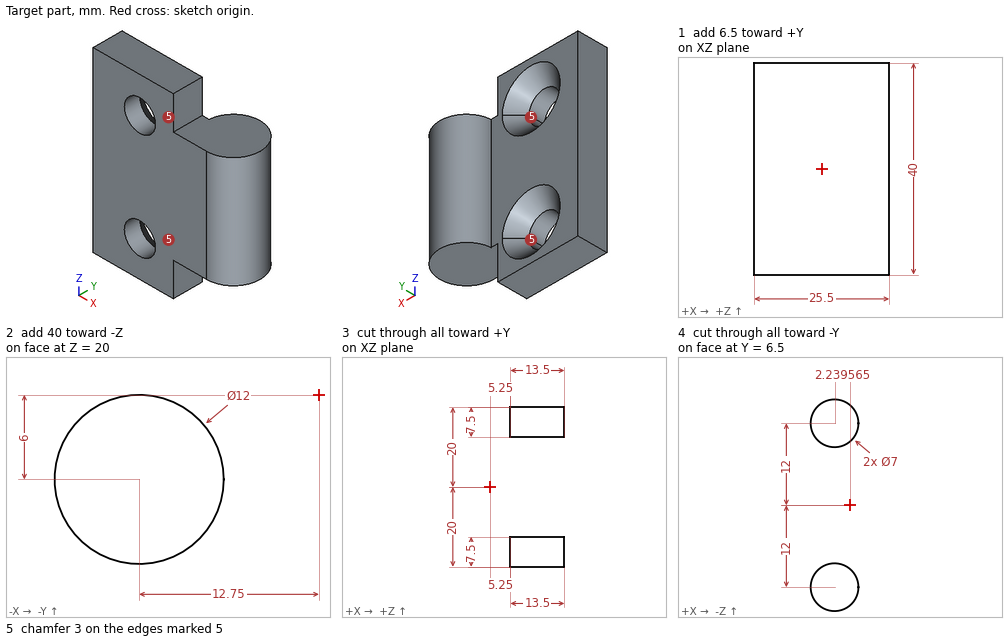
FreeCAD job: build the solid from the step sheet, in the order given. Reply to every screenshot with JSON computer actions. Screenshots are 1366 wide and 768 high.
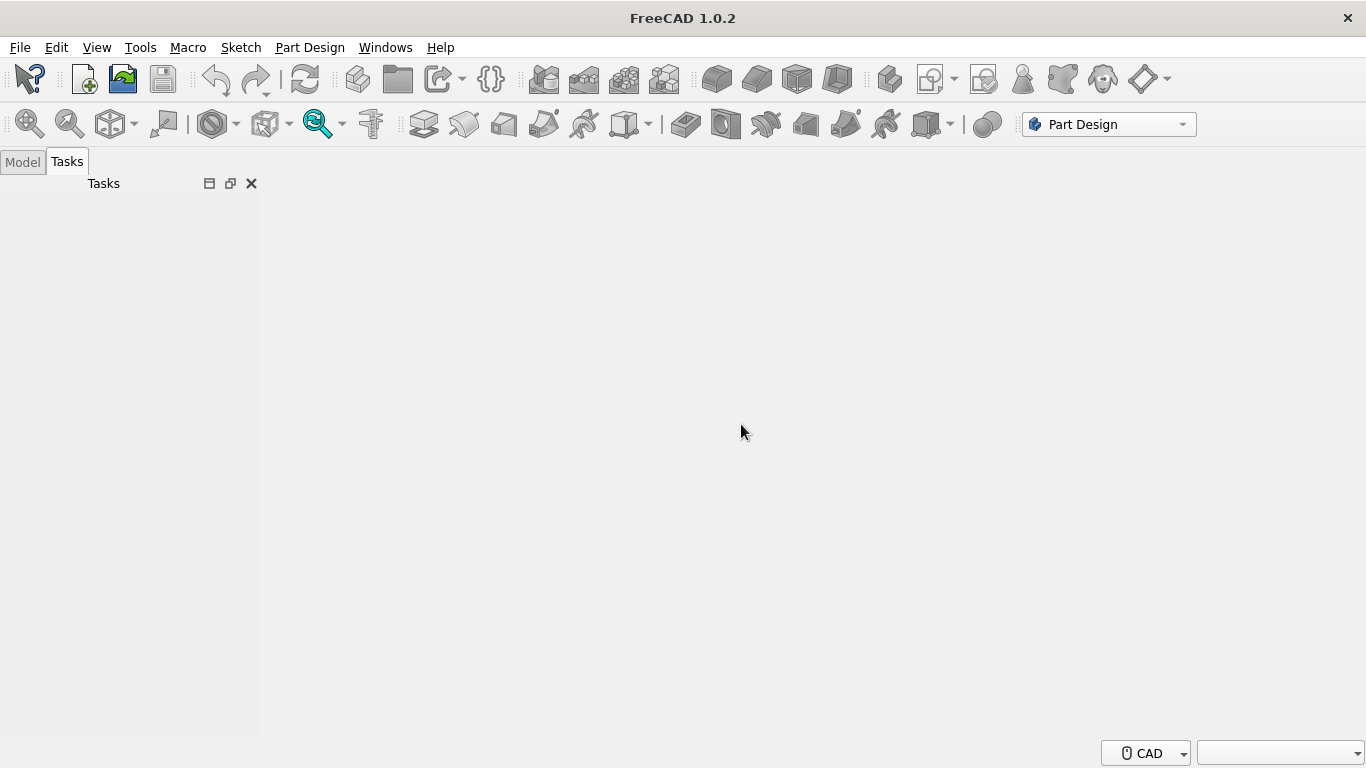
{"action": "key", "text": "ctrl+n"}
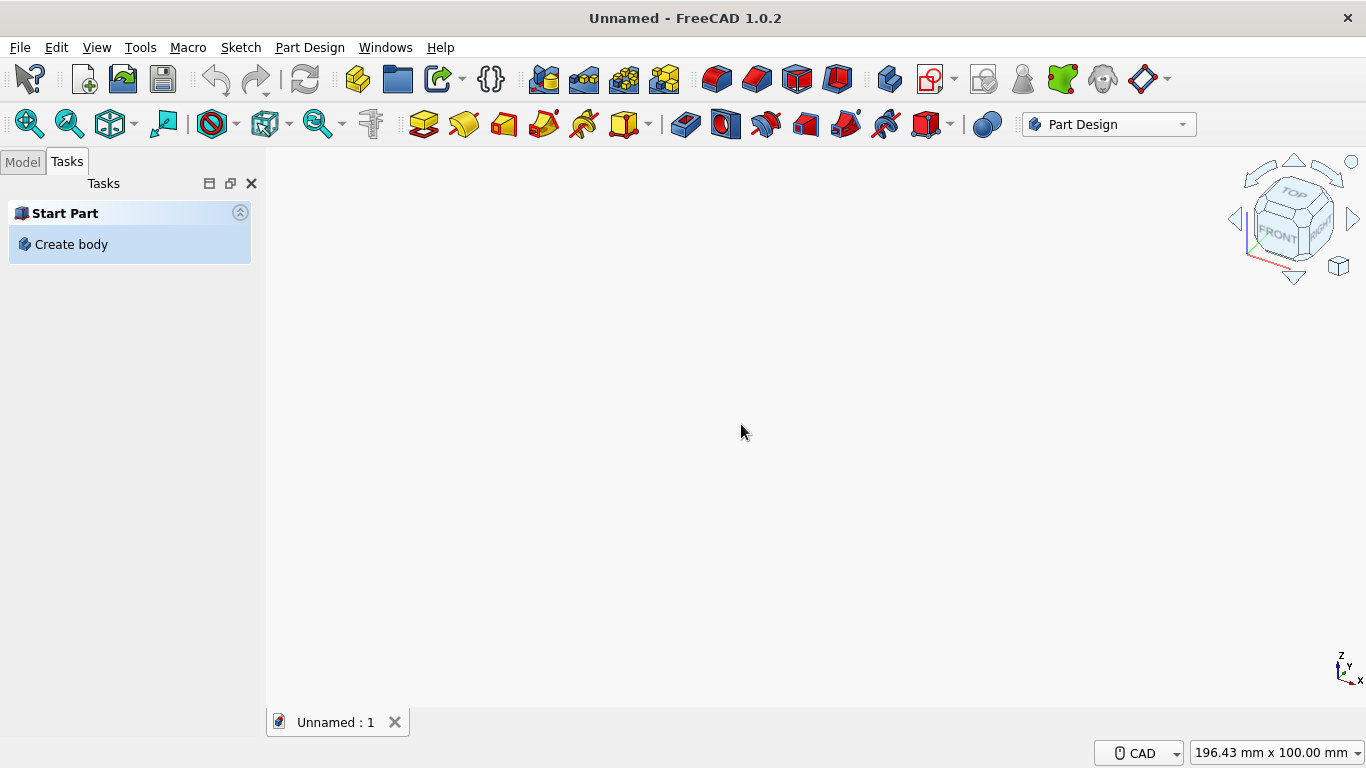
{"action": "left_click", "coordinate": [930, 80]}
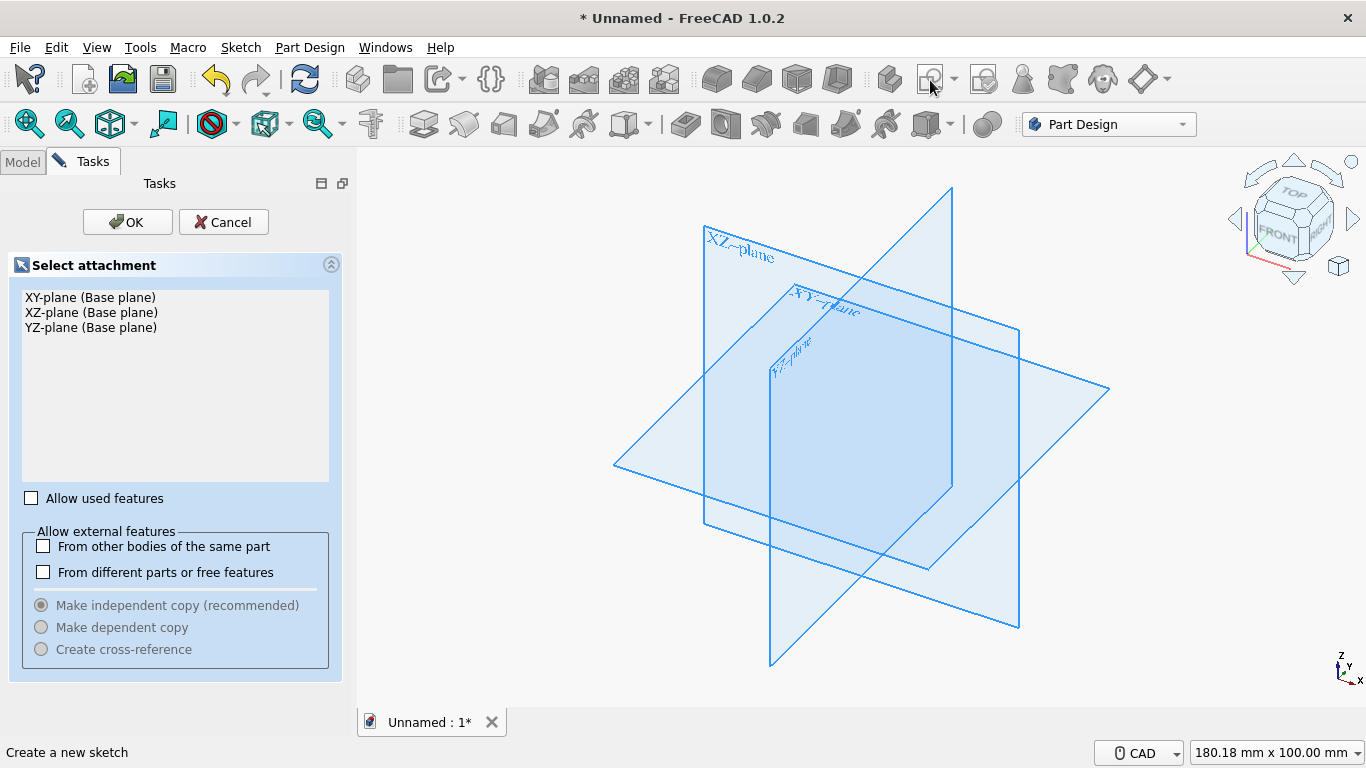
{"action": "left_click", "coordinate": [82, 312]}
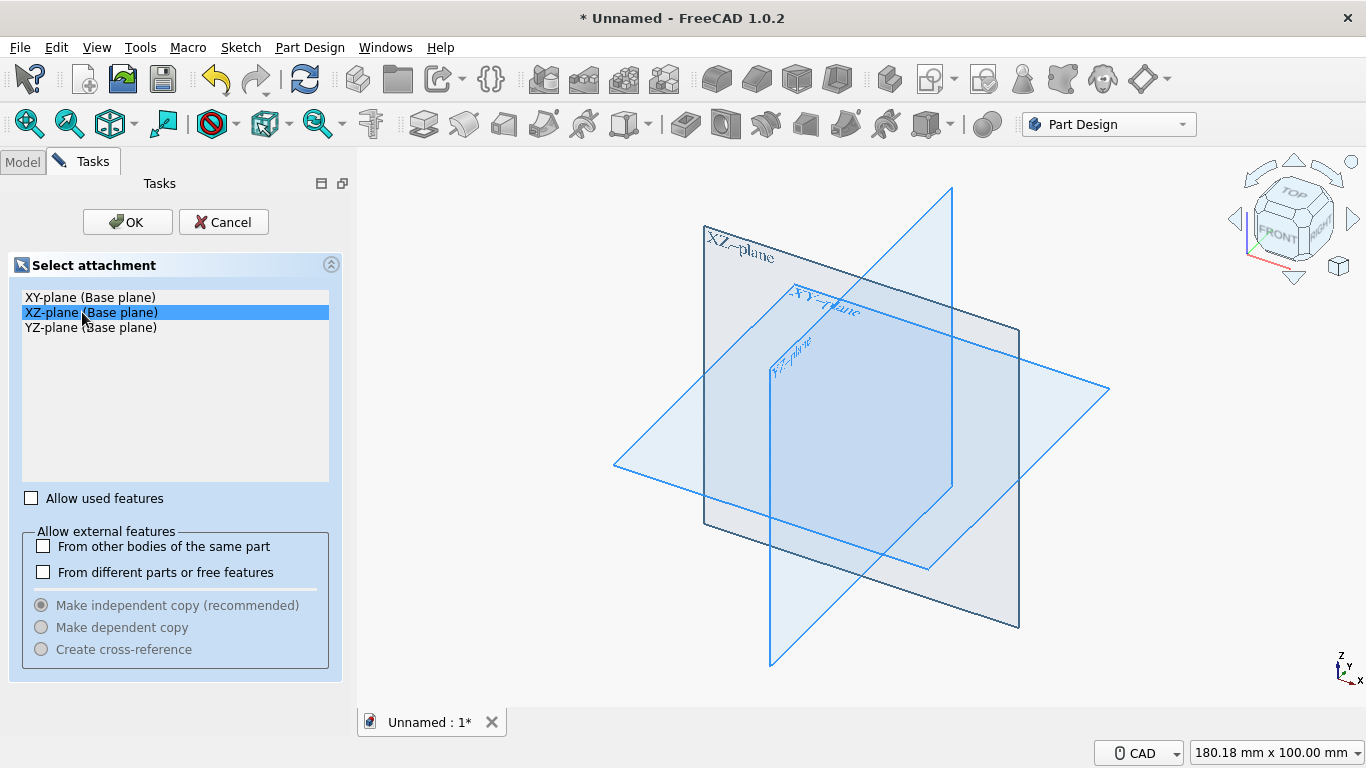
{"action": "left_click", "coordinate": [128, 222]}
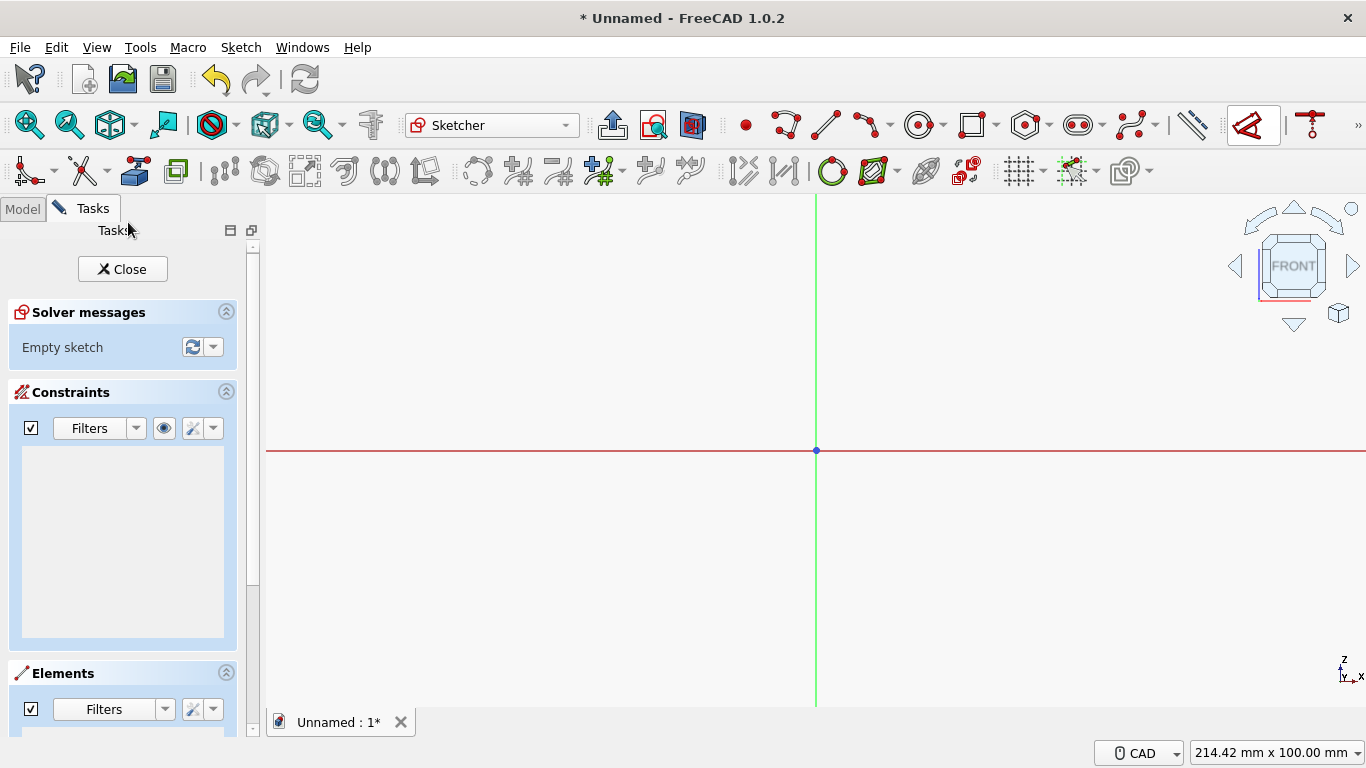
{"action": "scroll", "coordinate": [955, 451], "scroll_direction": "up", "scroll_amount": 2}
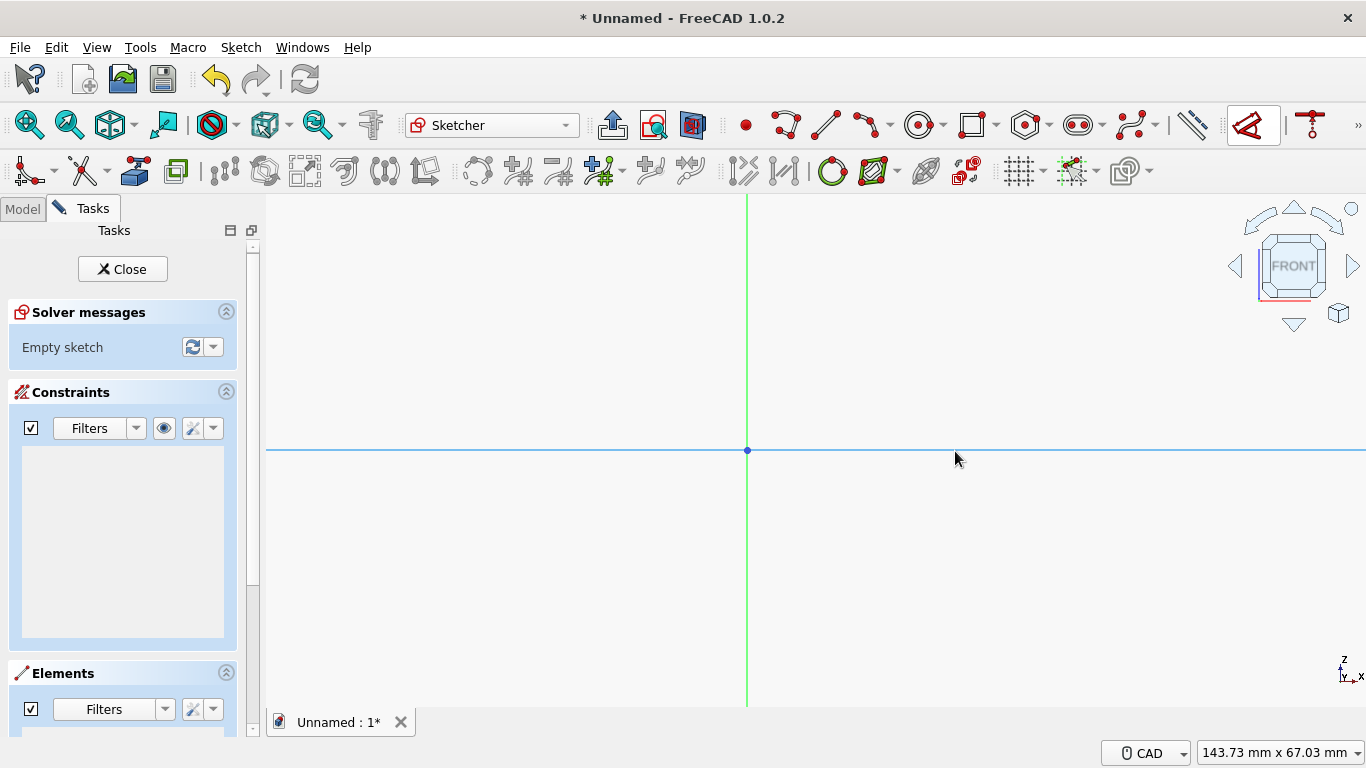
{"action": "key", "text": "g v"}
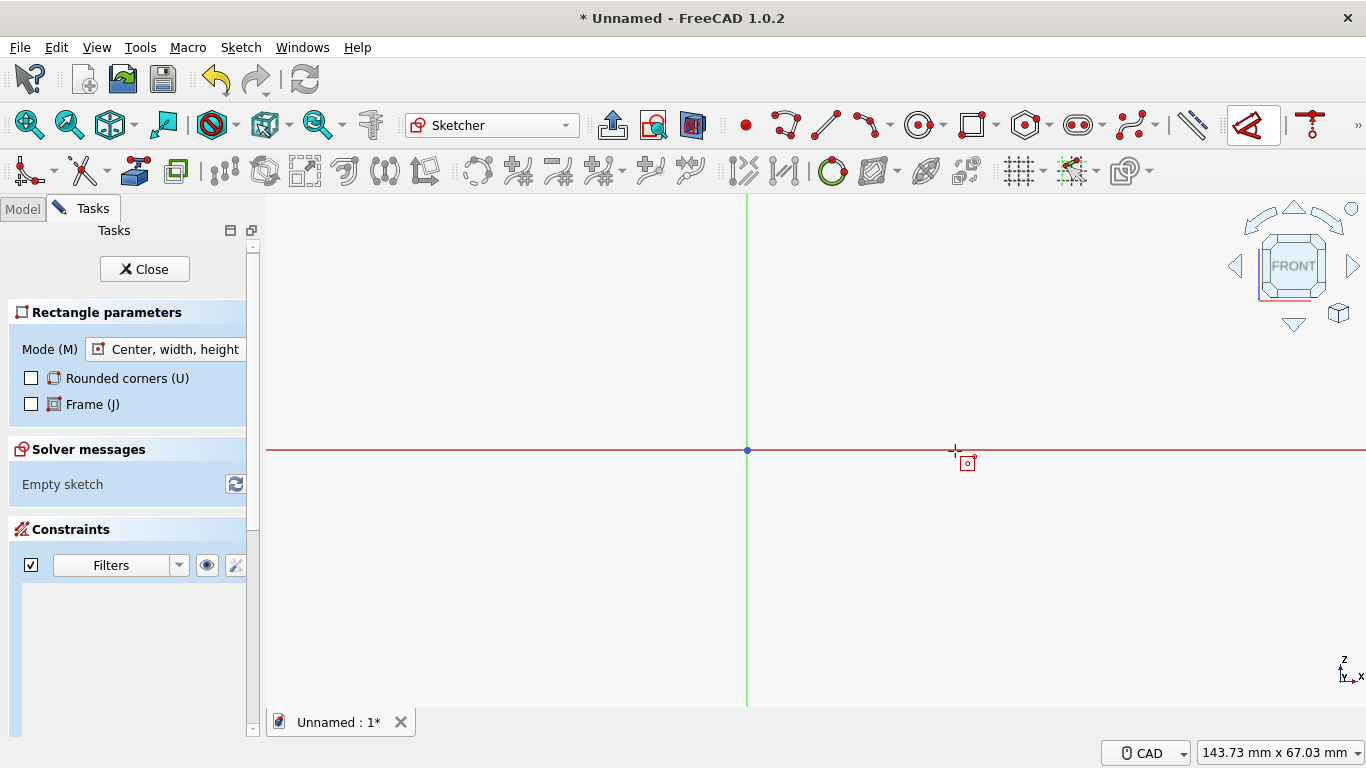
{"action": "left_click", "coordinate": [747, 450]}
{"action": "left_click", "coordinate": [845, 297]}
{"action": "key", "text": "Escape"}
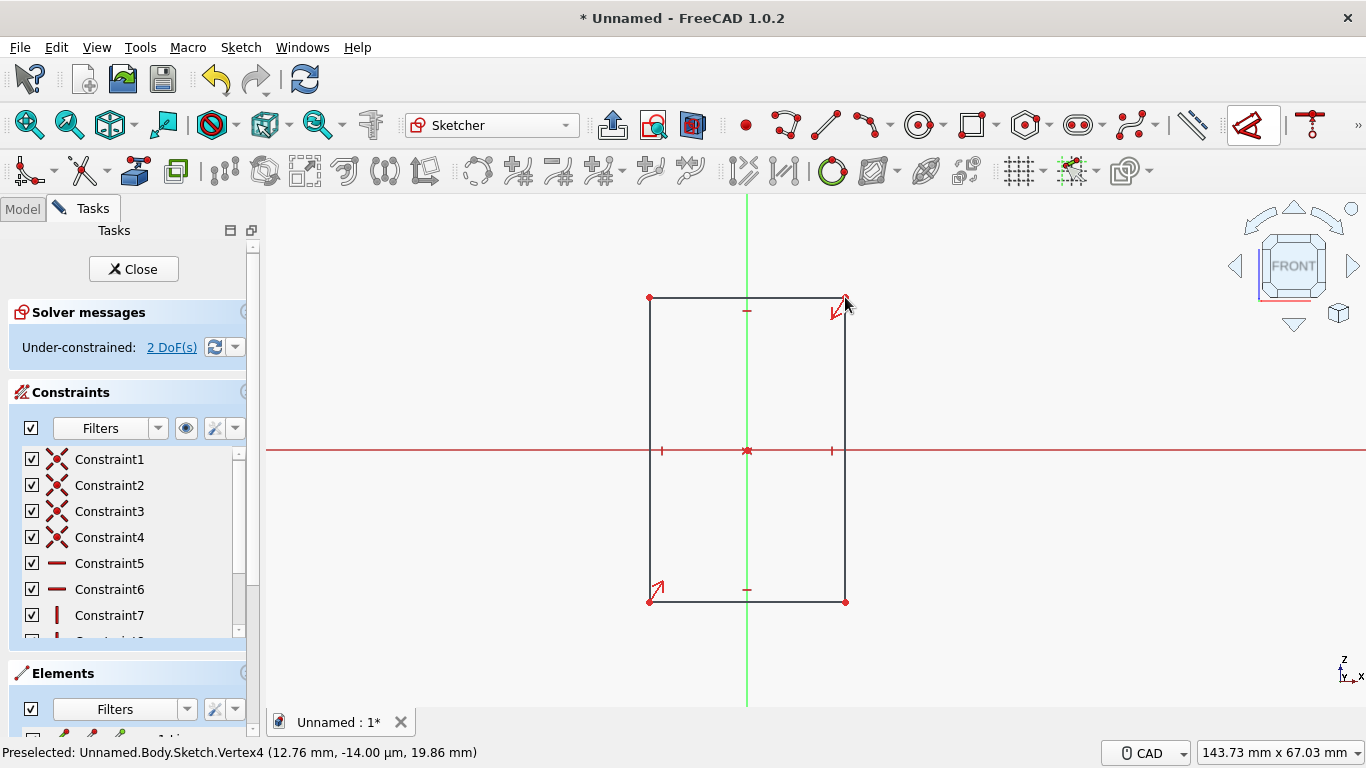
{"action": "key", "text": "d"}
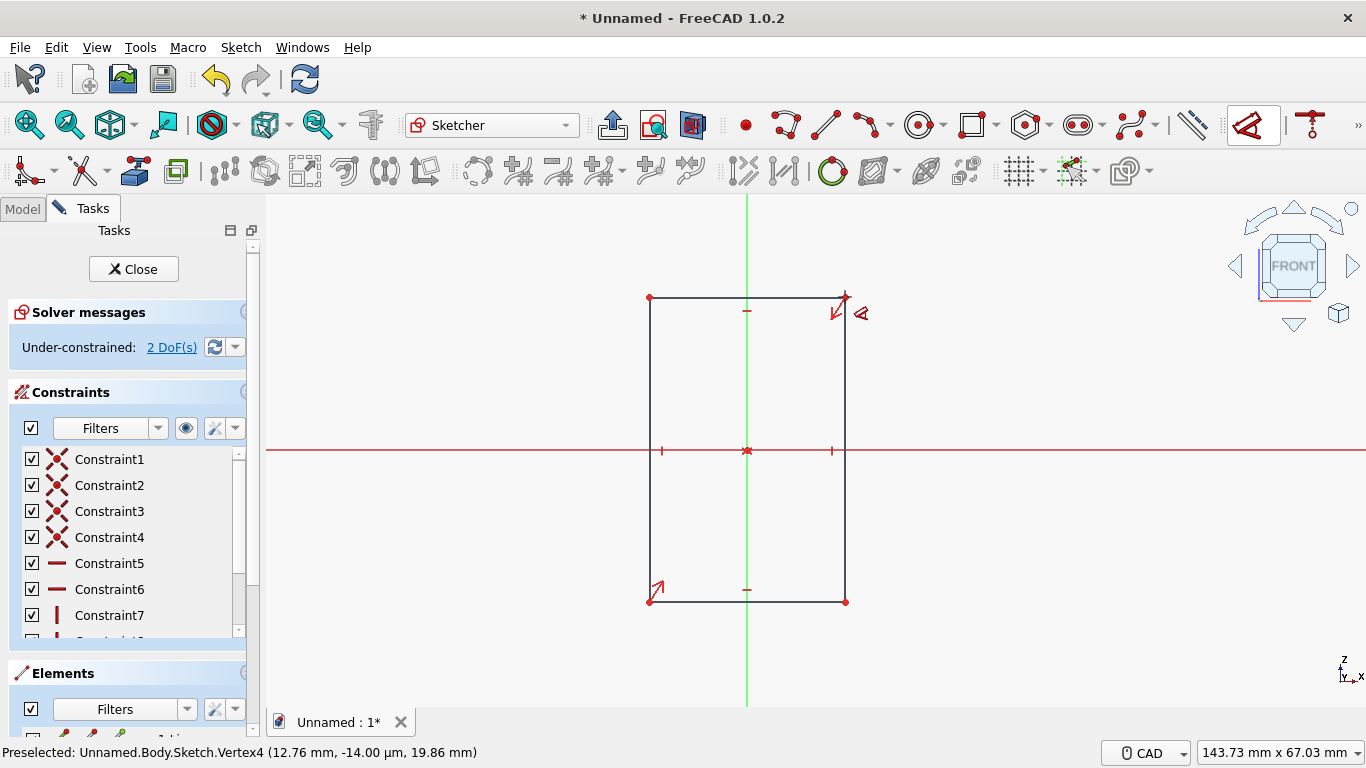
{"action": "left_click", "coordinate": [845, 511]}
{"action": "left_click", "coordinate": [879, 380]}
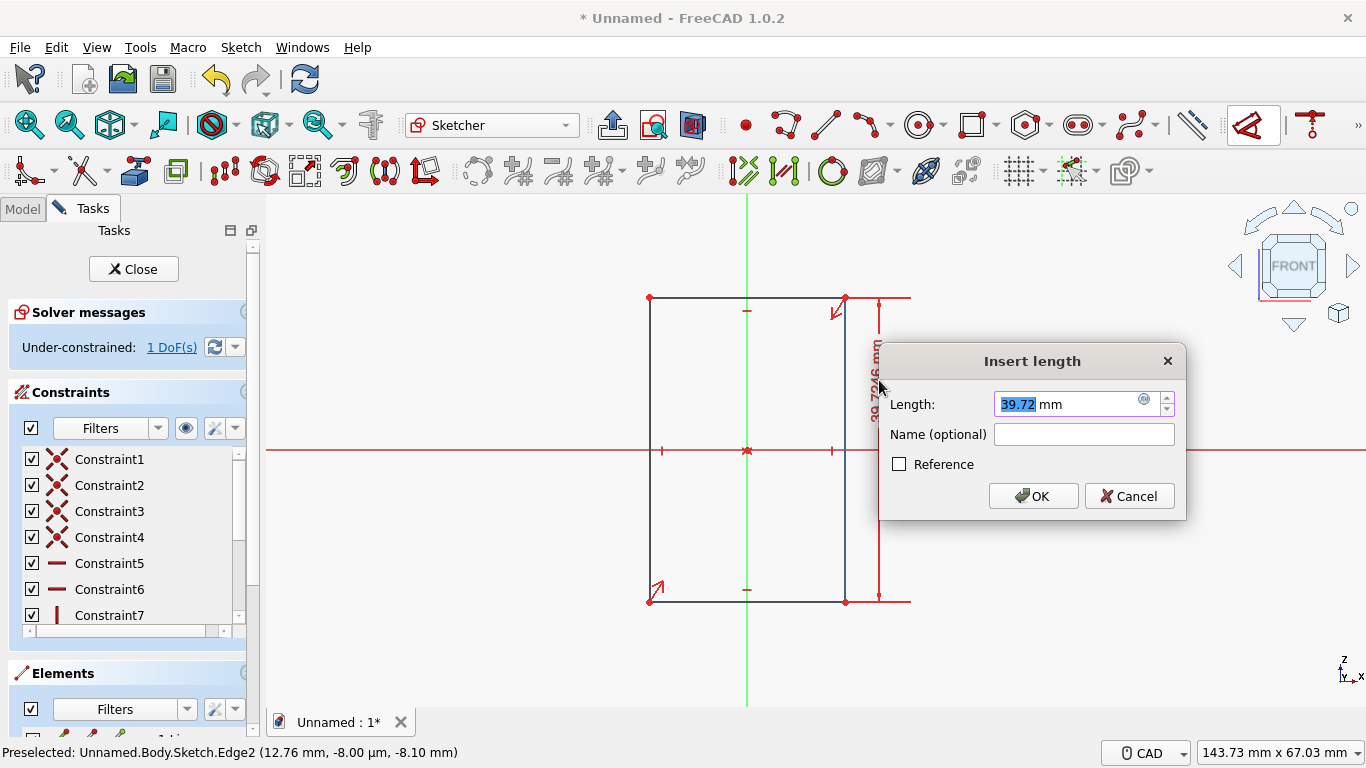
{"action": "type", "text": "40"}
{"action": "key", "text": "Return"}